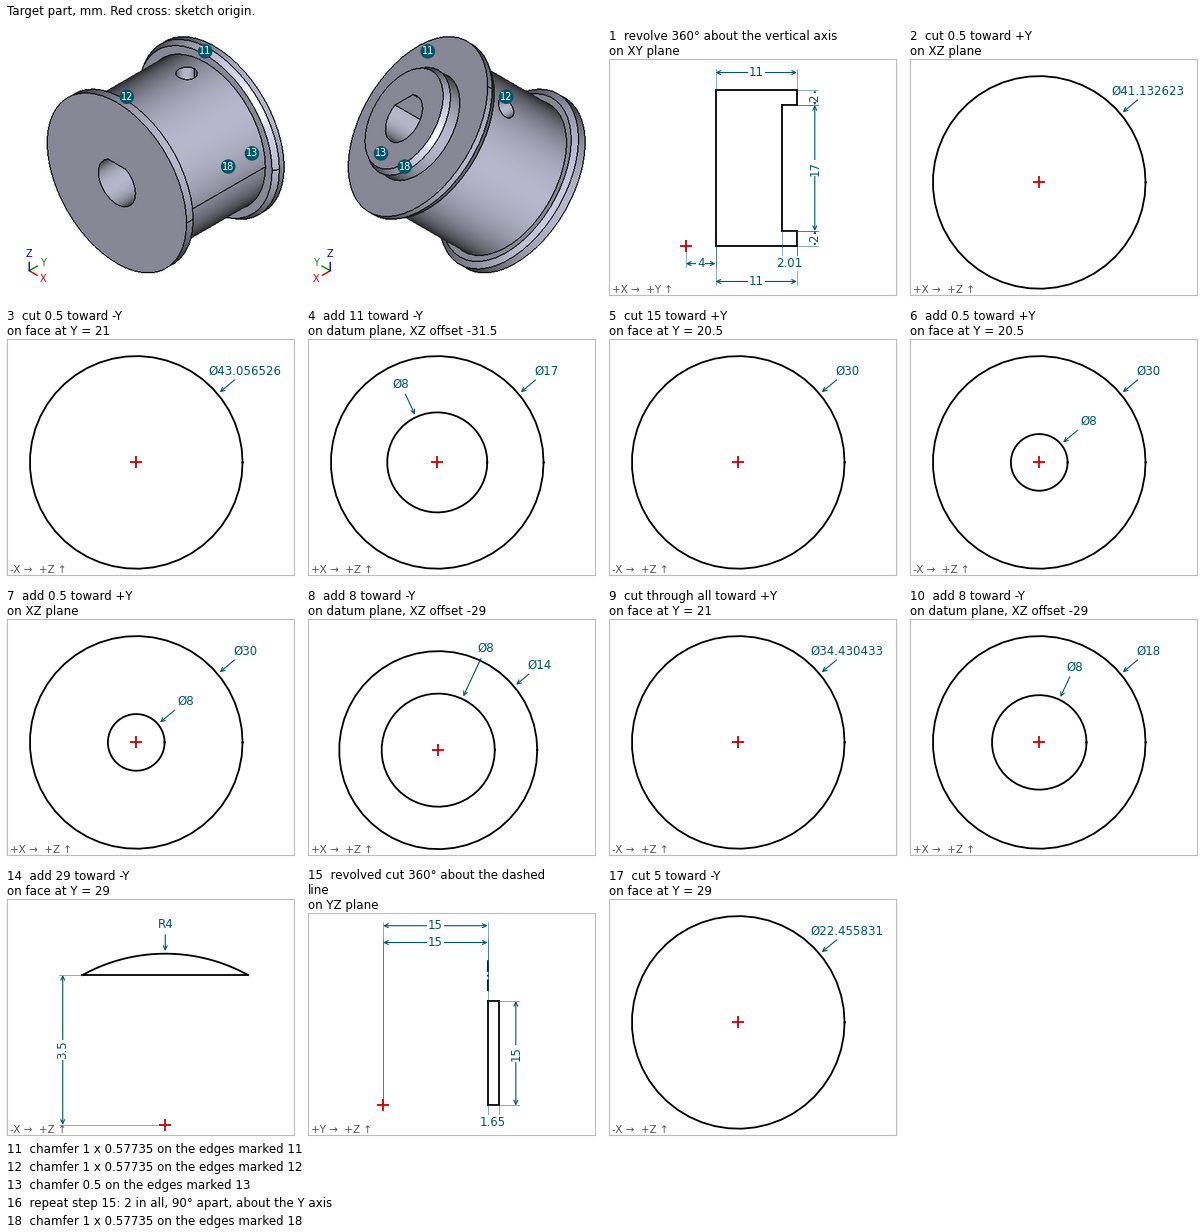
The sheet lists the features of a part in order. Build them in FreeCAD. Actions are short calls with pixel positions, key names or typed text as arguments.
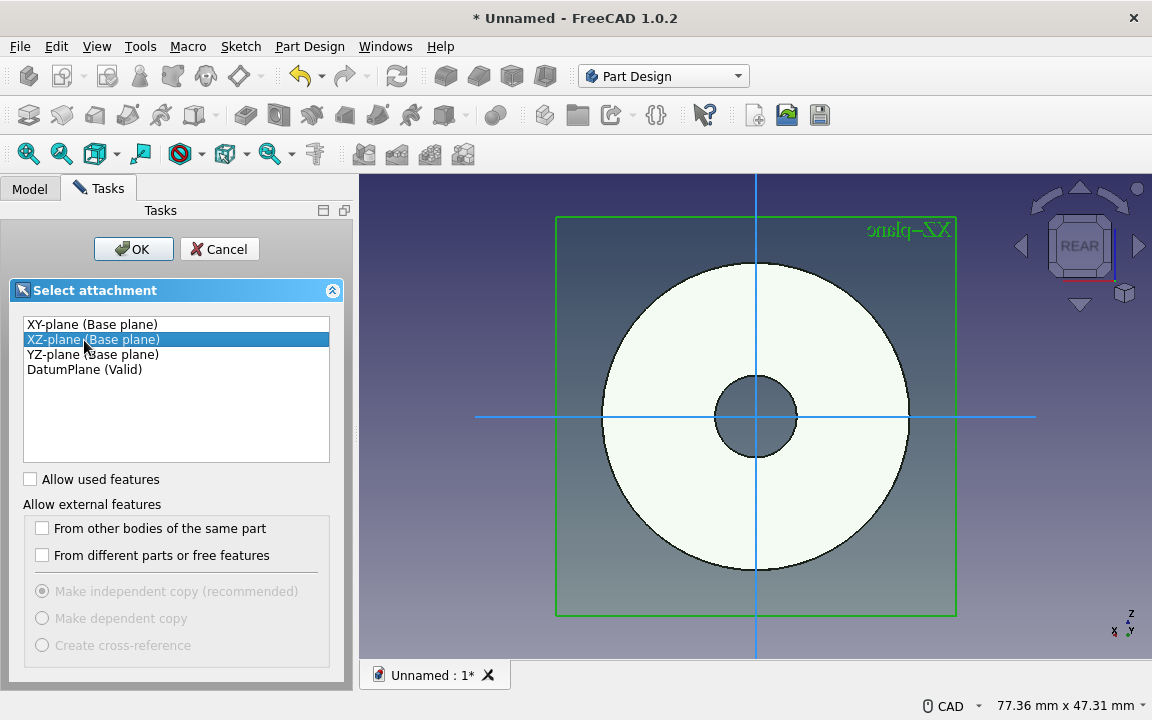
click(134, 249)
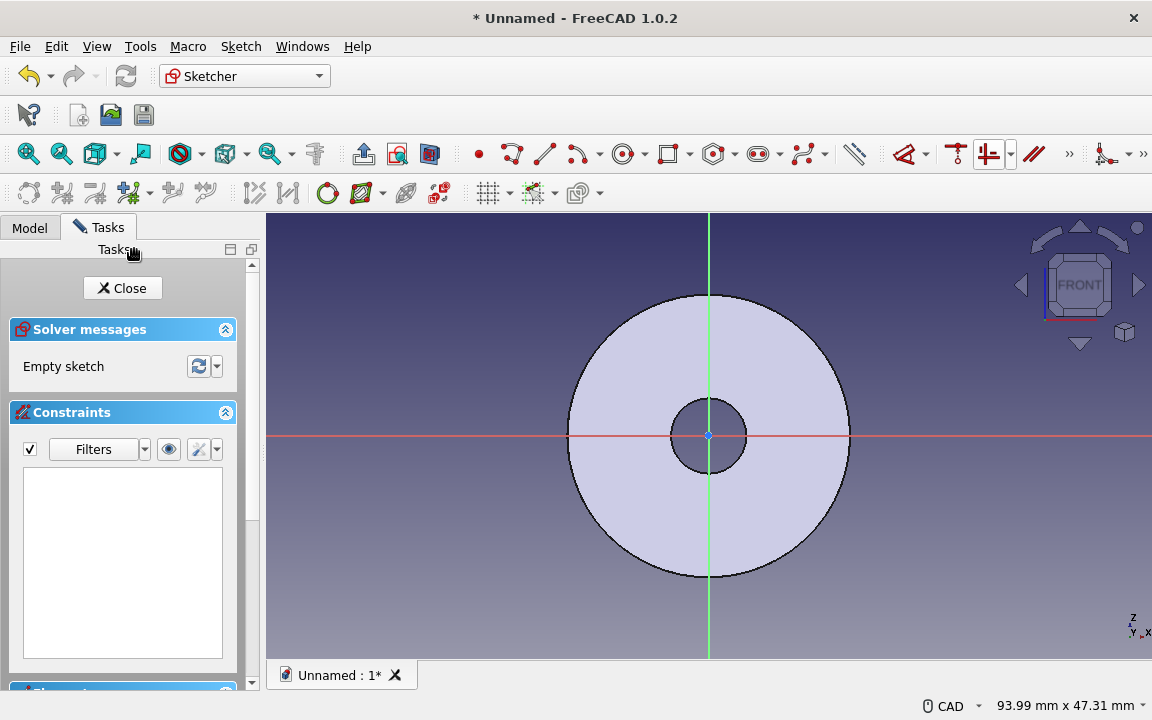
click(622, 154)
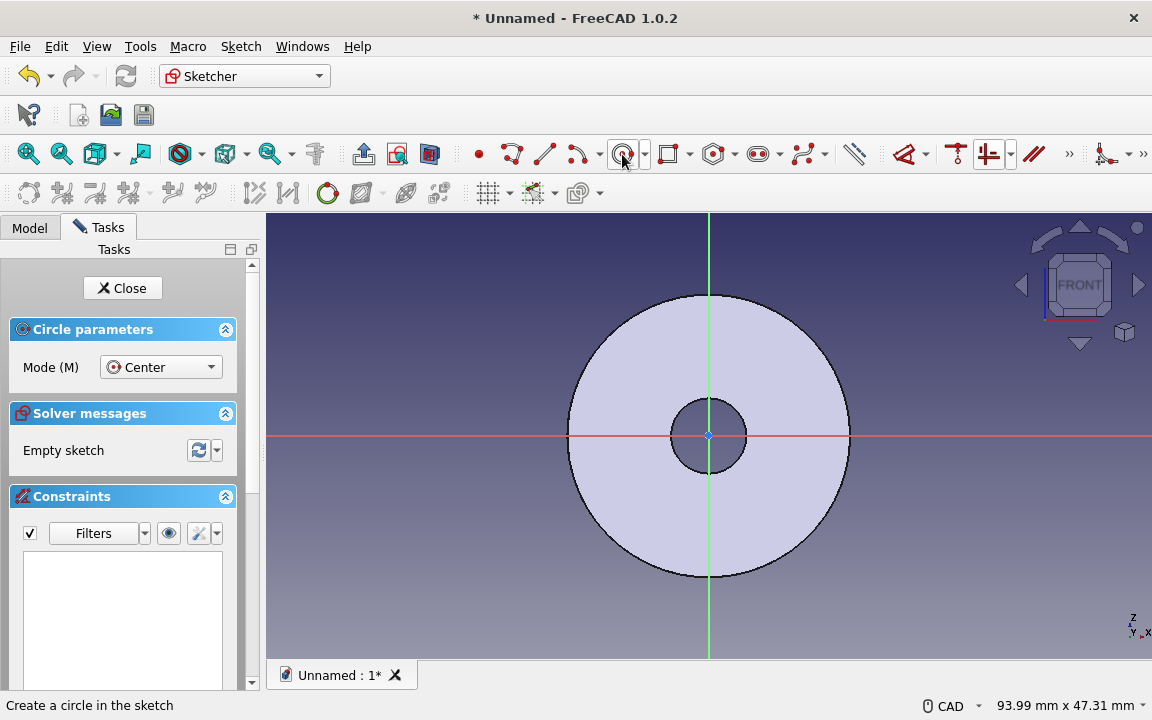
click(709, 436)
move(809, 336)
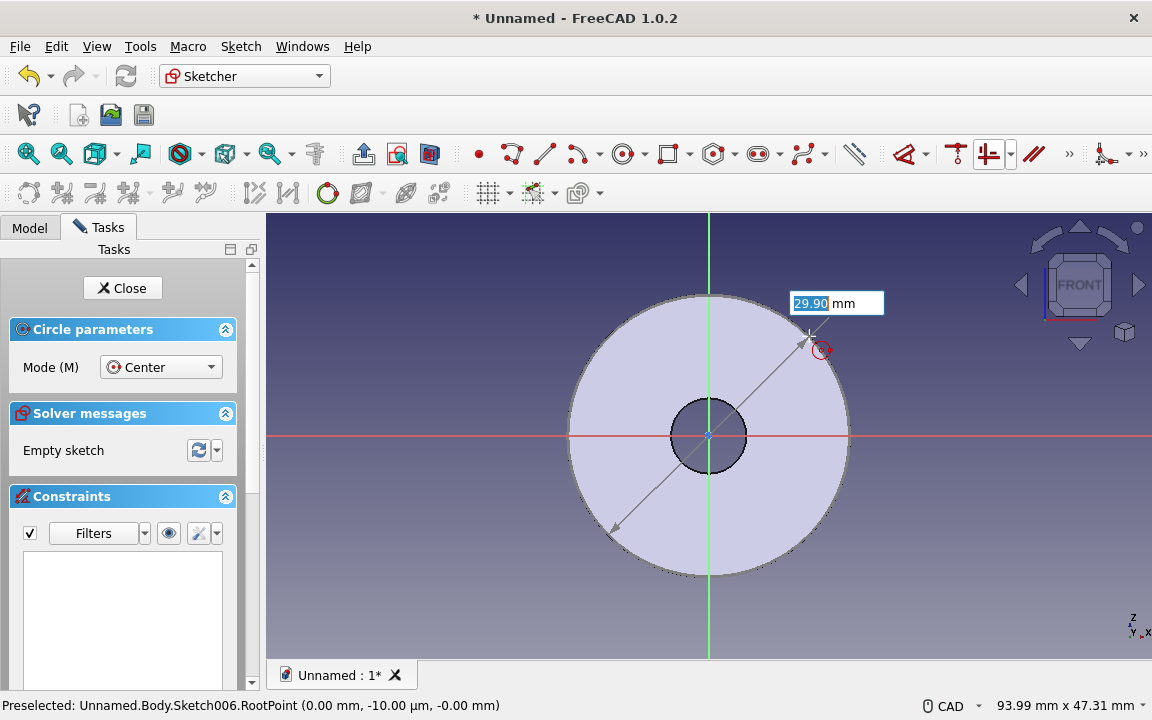
text(30)
key(Return)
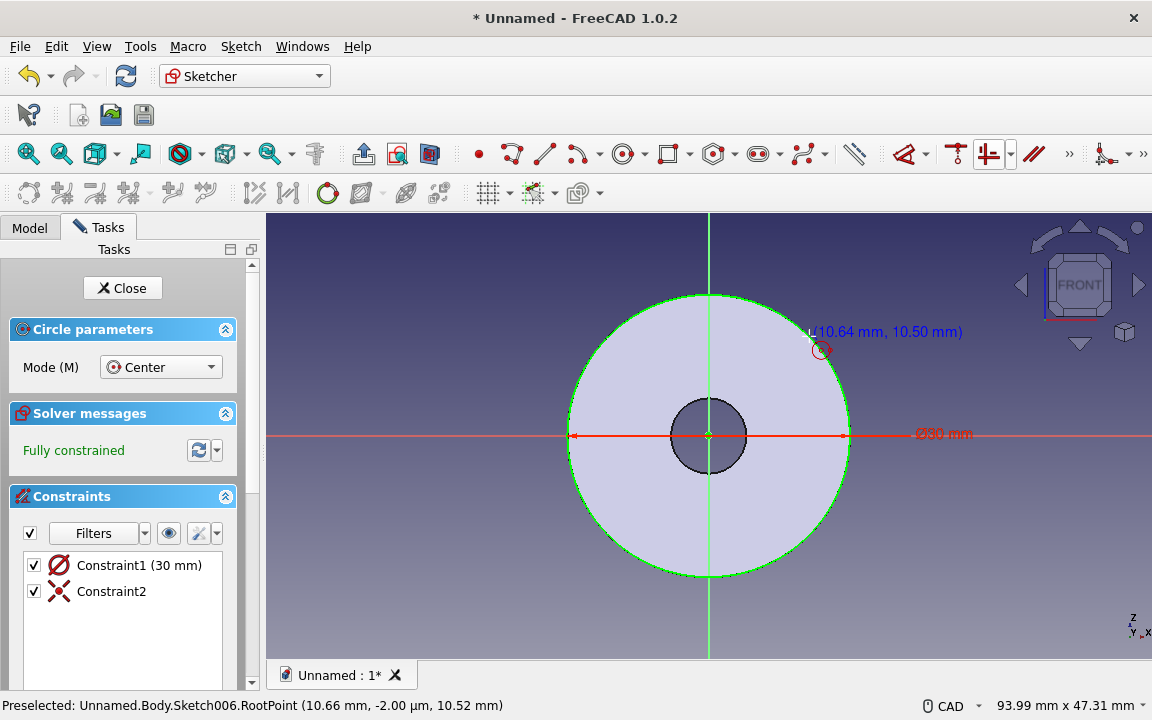
click(709, 436)
move(735, 409)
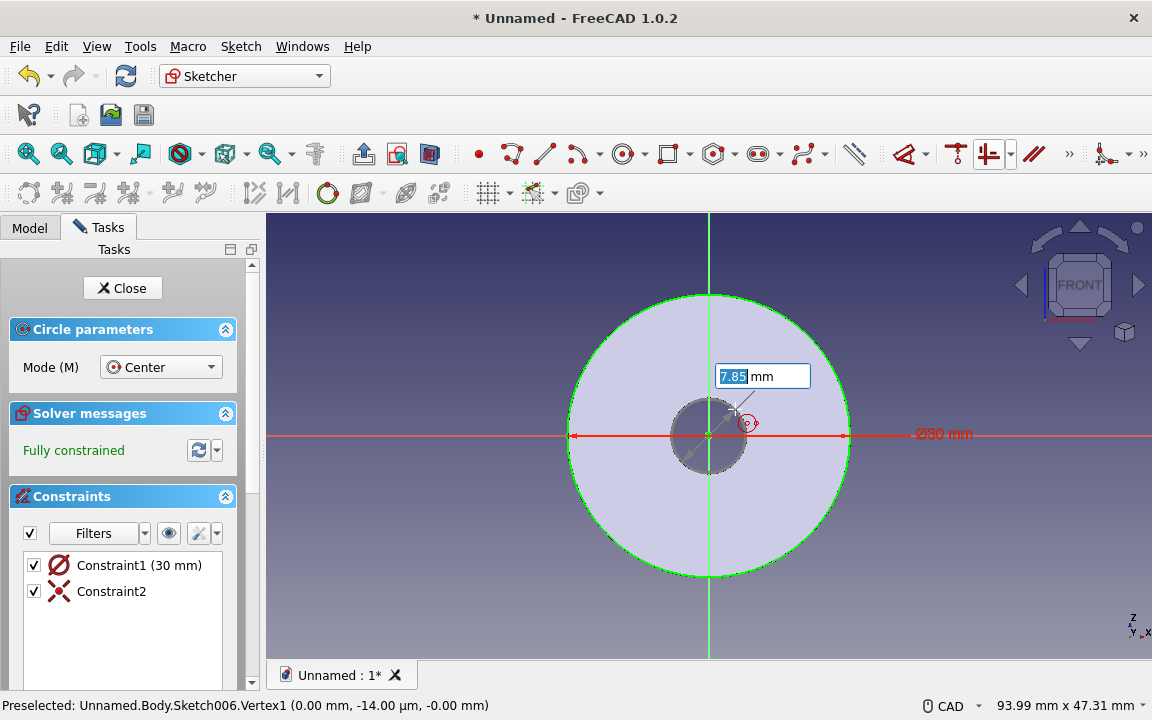
text(8)
key(Return)
key(Escape)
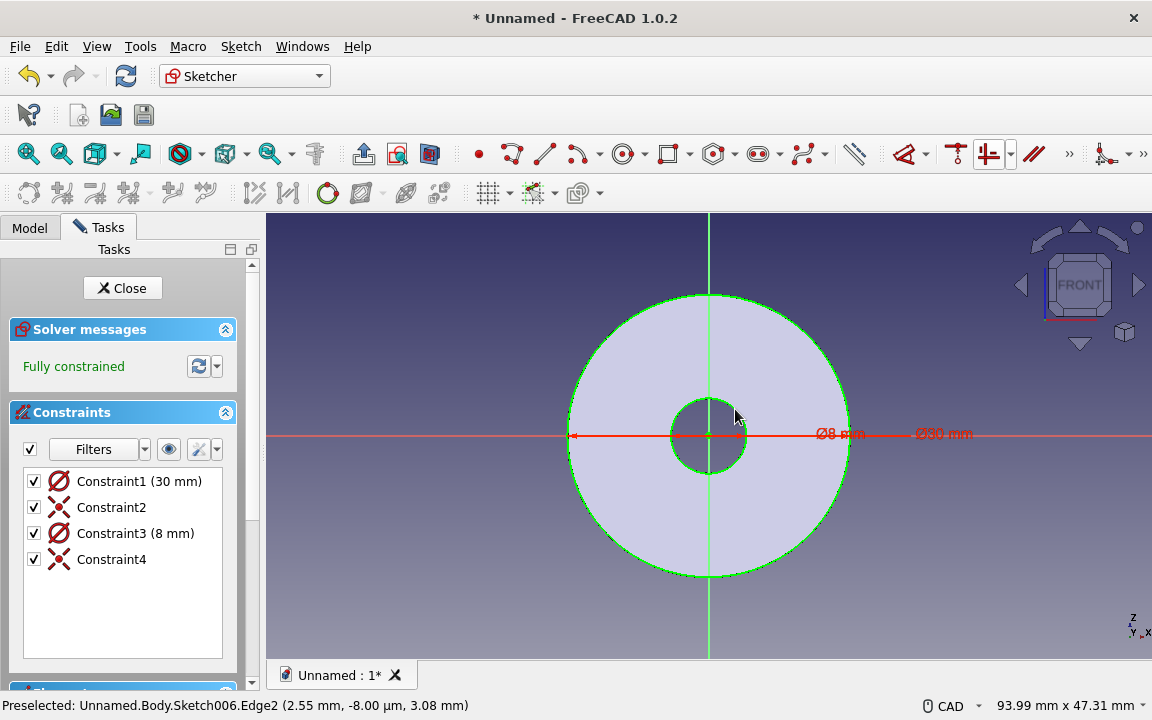
click(123, 288)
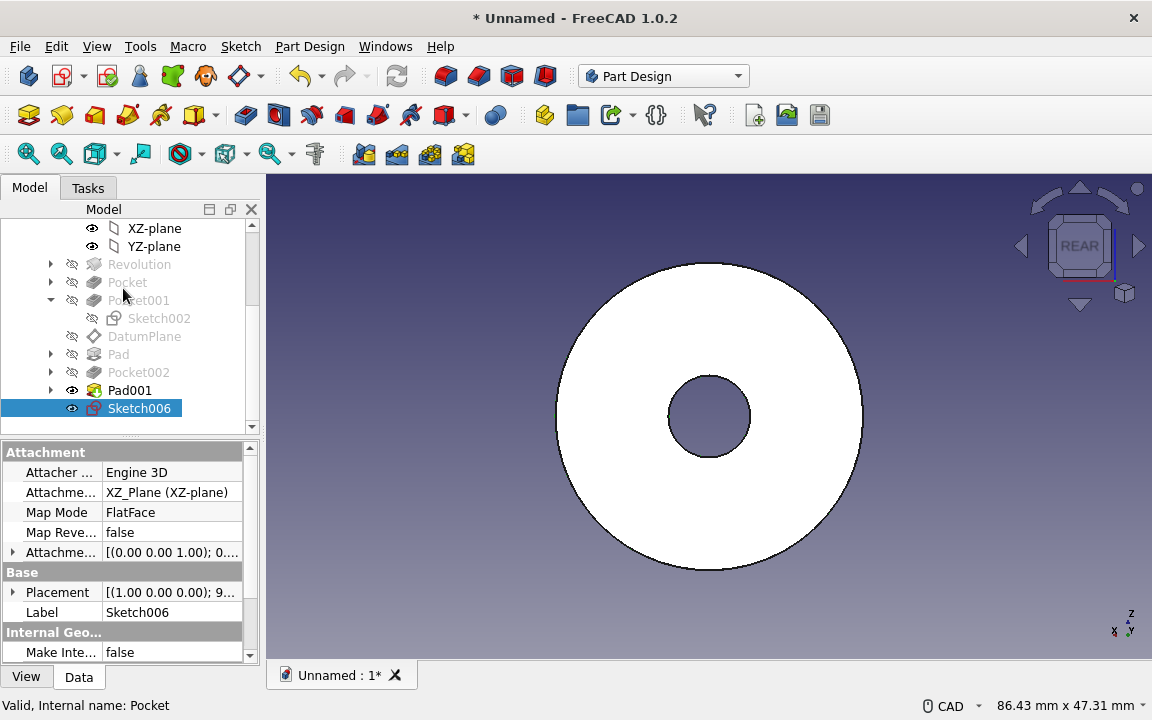
click(29, 116)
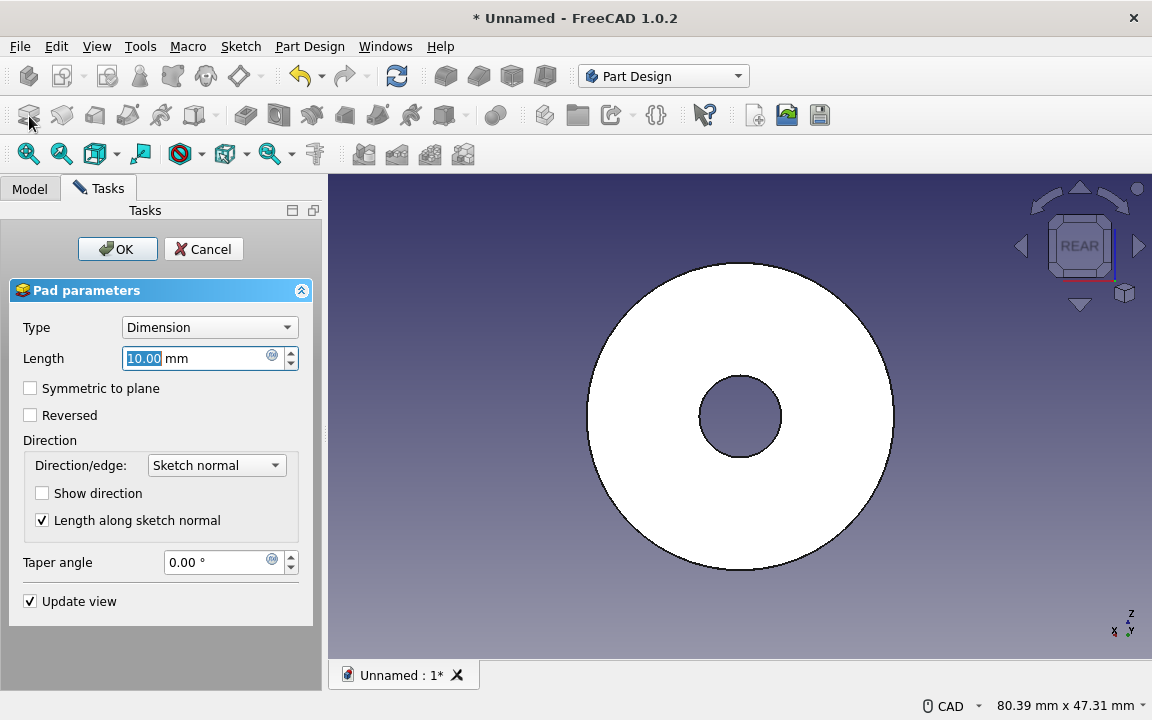
text(0.5)
key(Tab)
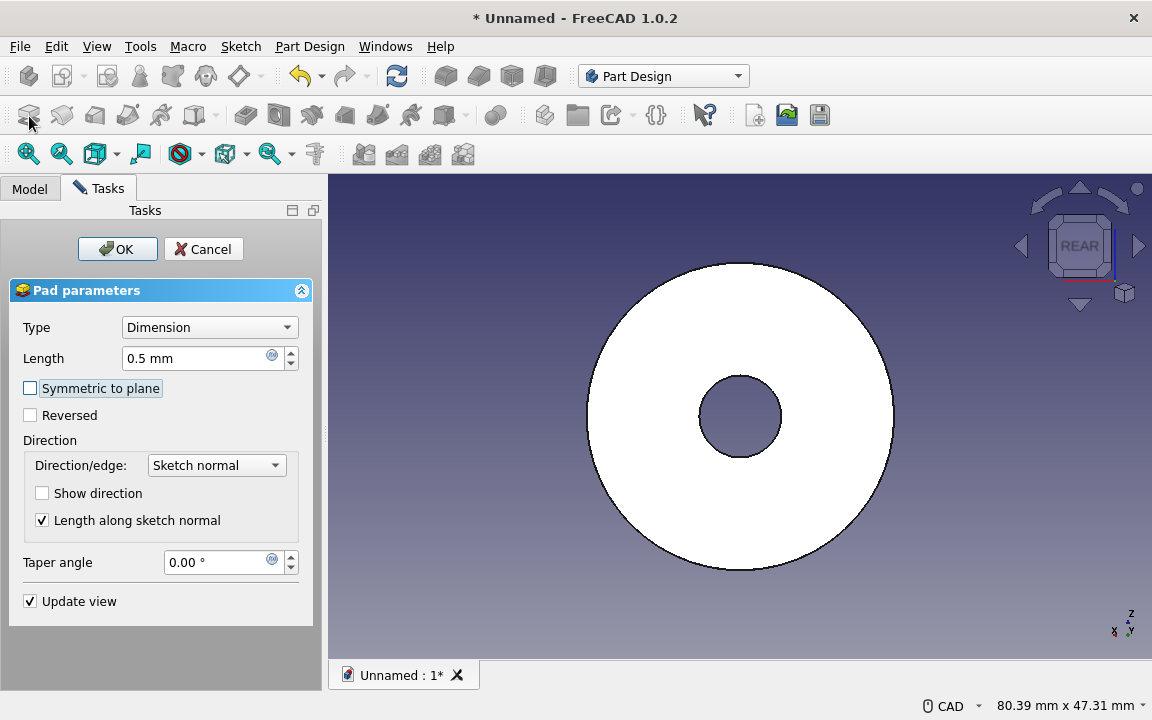
click(31, 415)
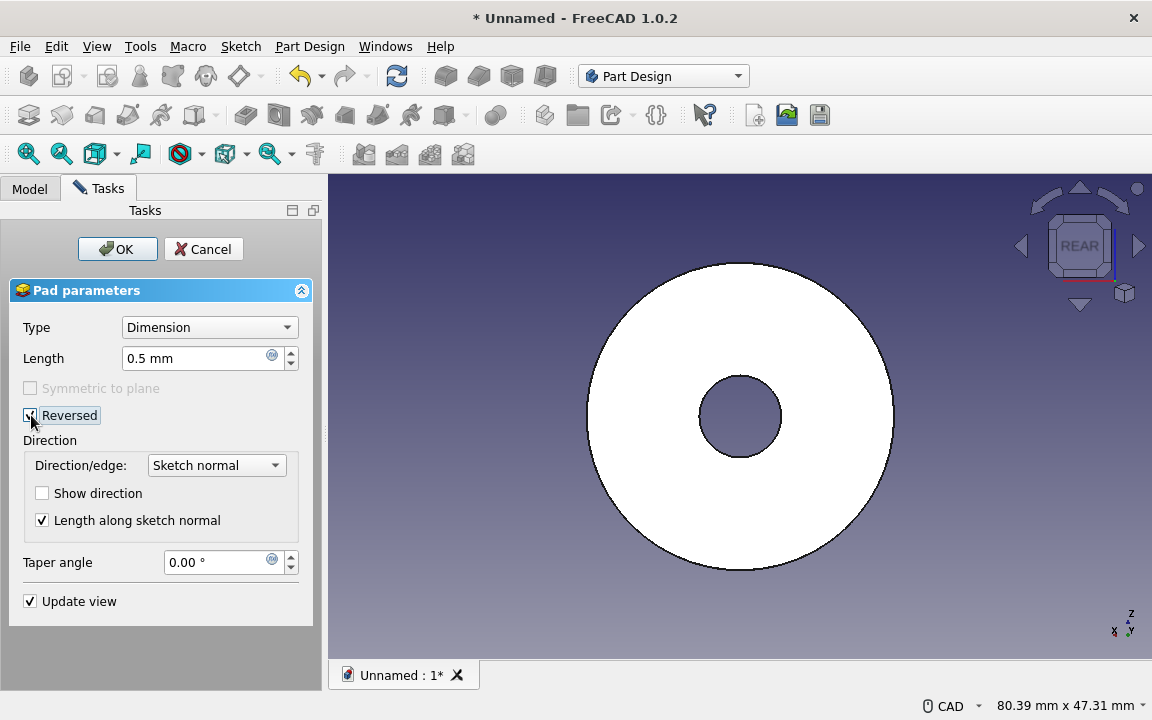
click(118, 249)